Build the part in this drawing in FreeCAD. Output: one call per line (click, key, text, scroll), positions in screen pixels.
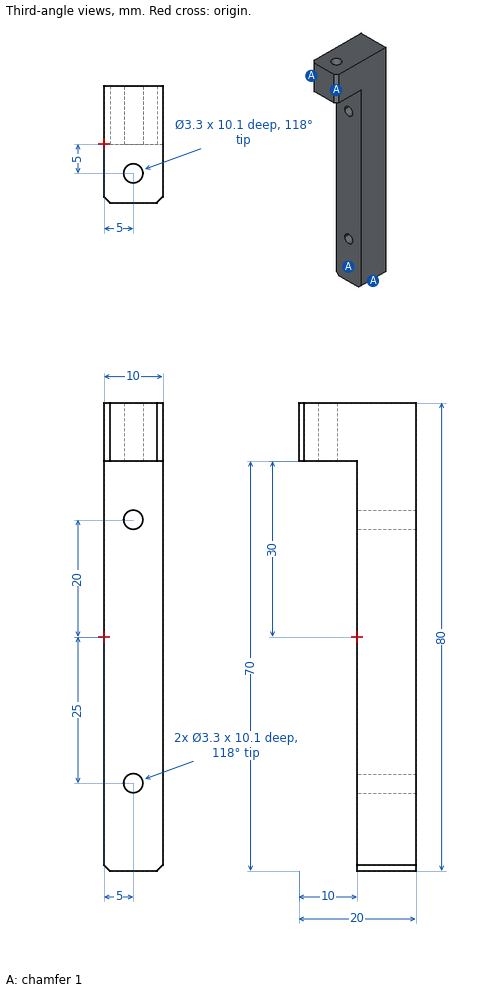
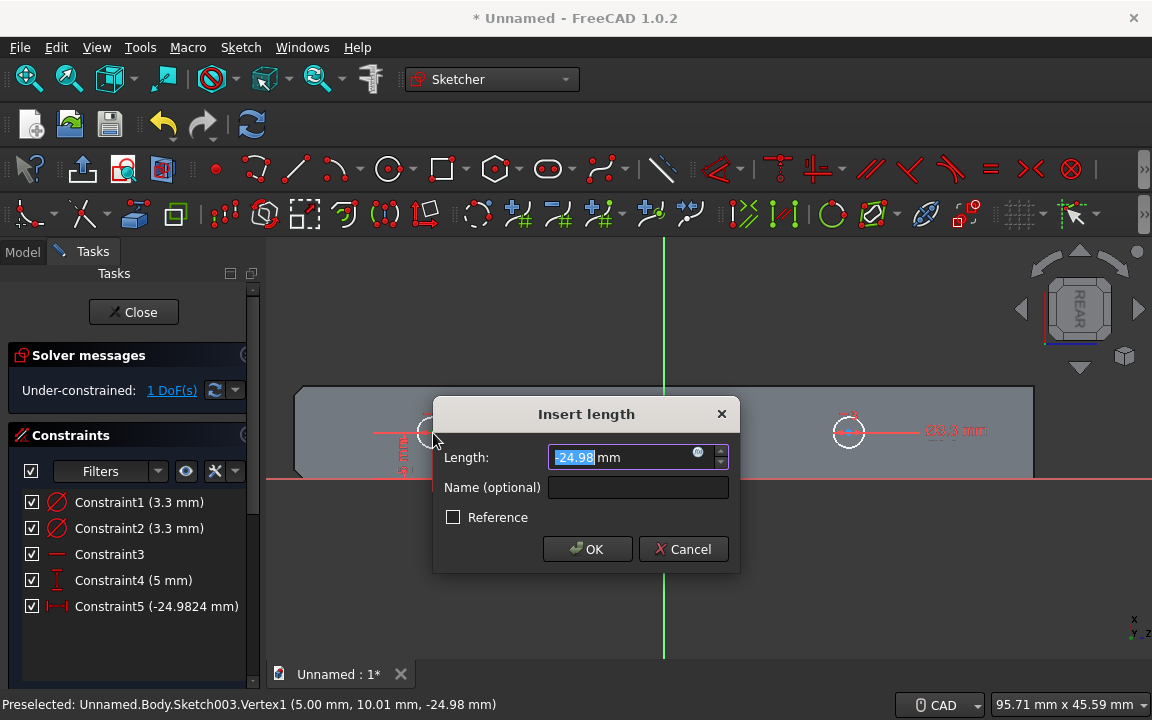
text(-25)
key(Return)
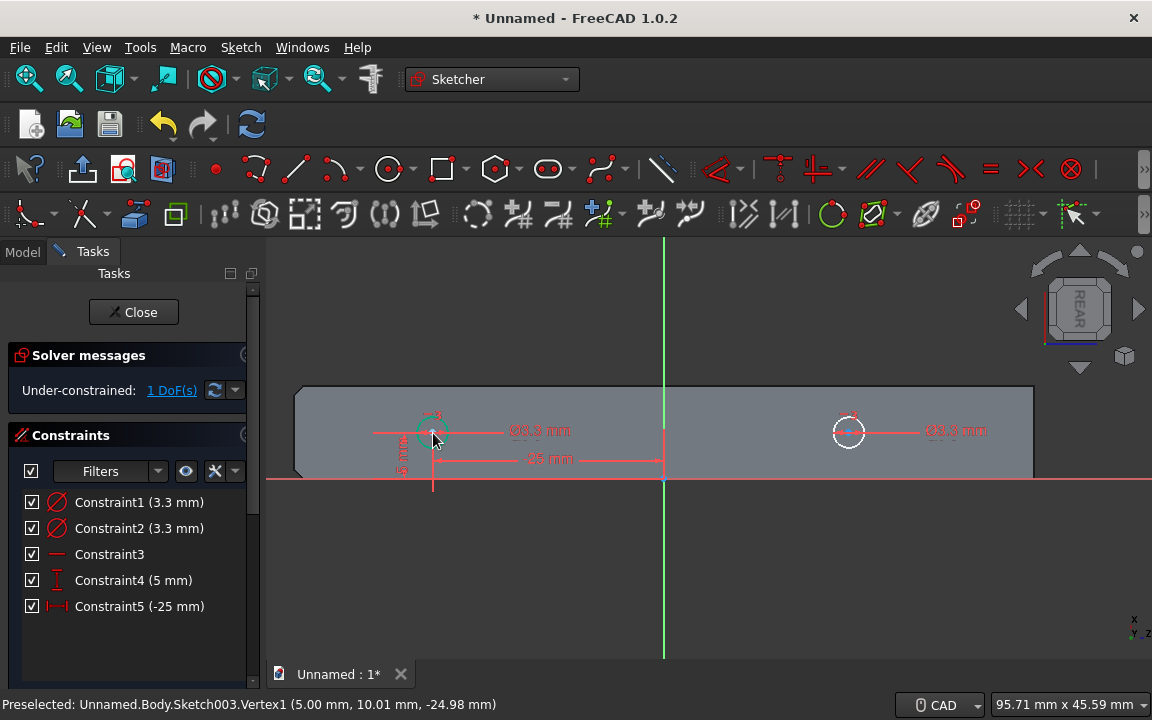
click(849, 433)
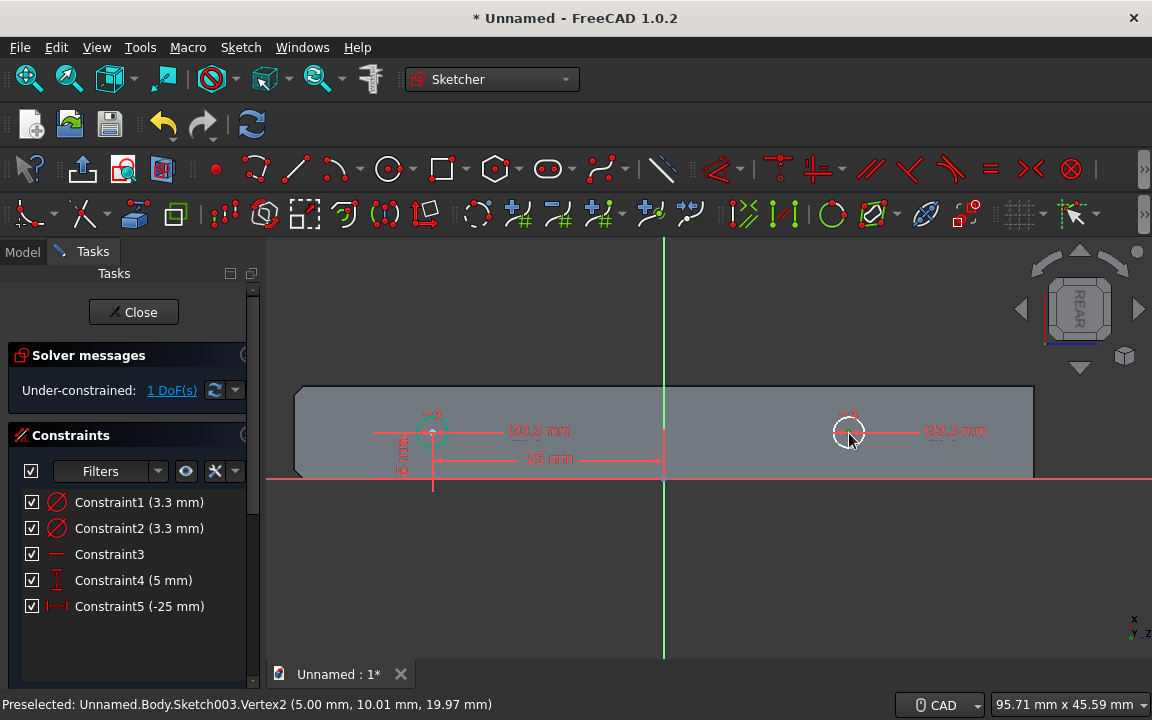
key(l)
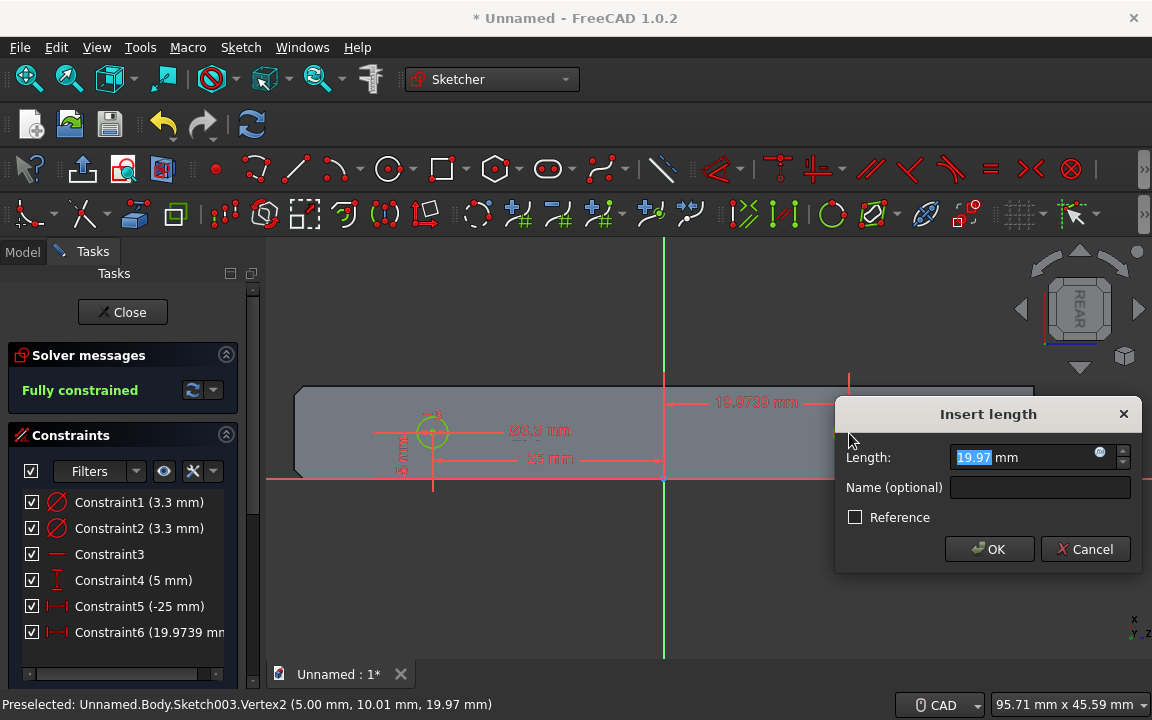
text(20)
key(Return)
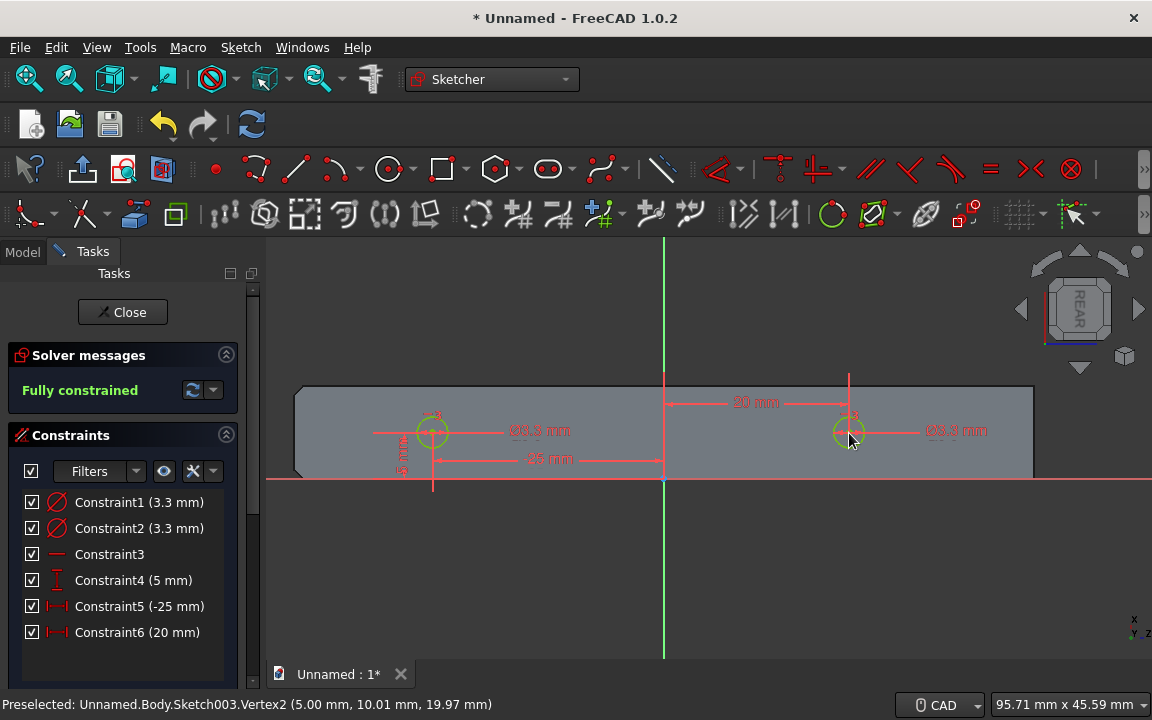
click(123, 312)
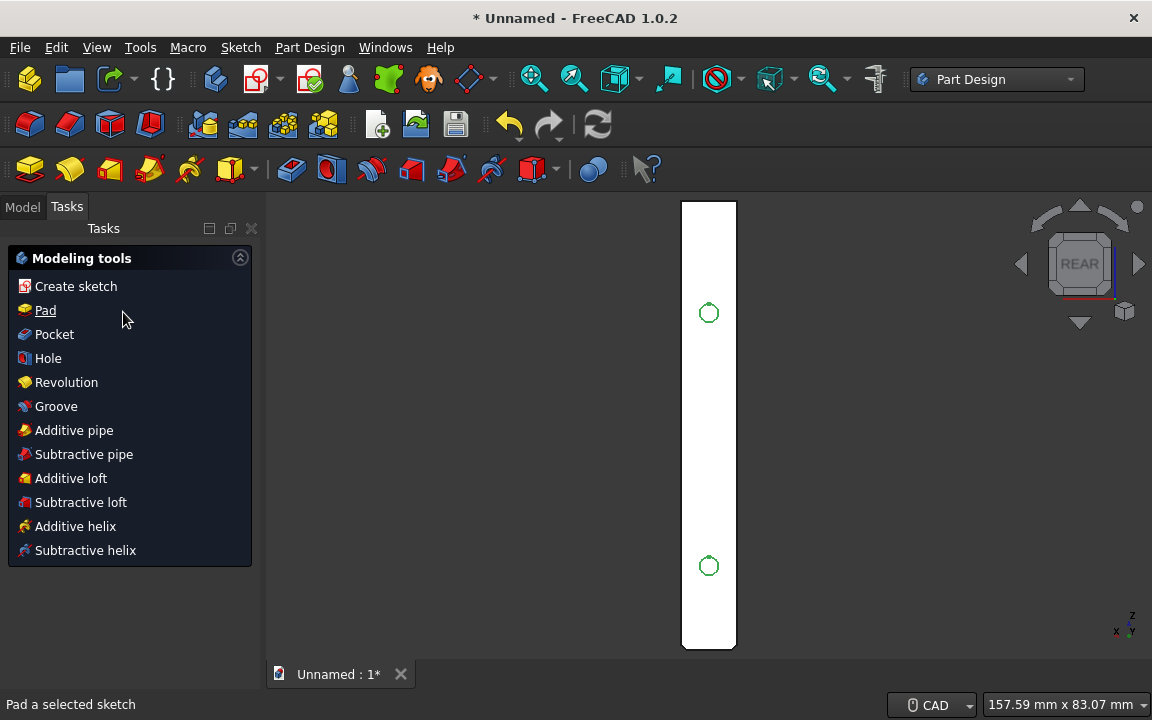
click(332, 170)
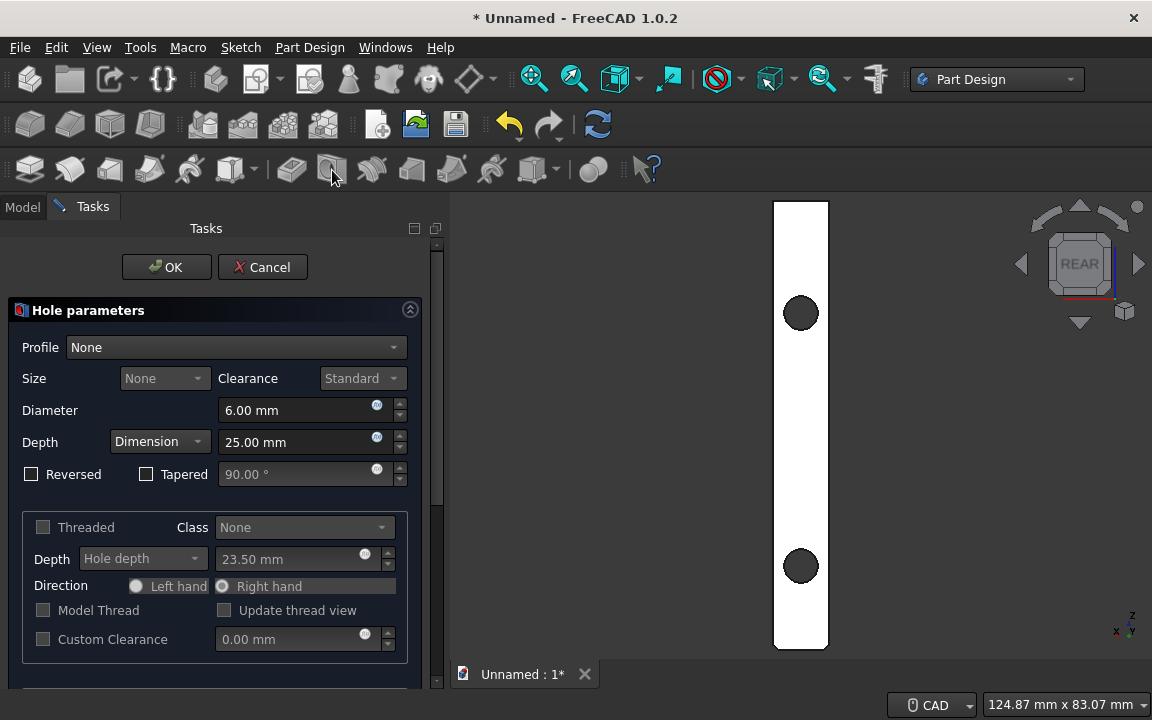
triple_click(305, 410)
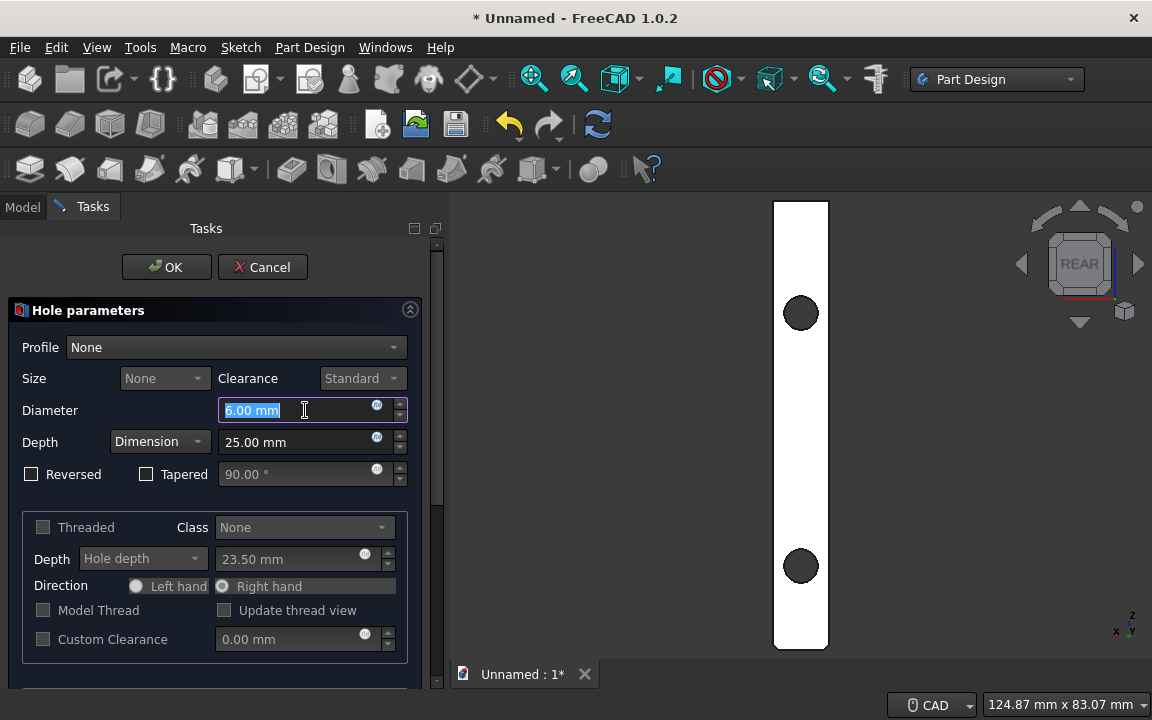
text(3.3)
key(Tab)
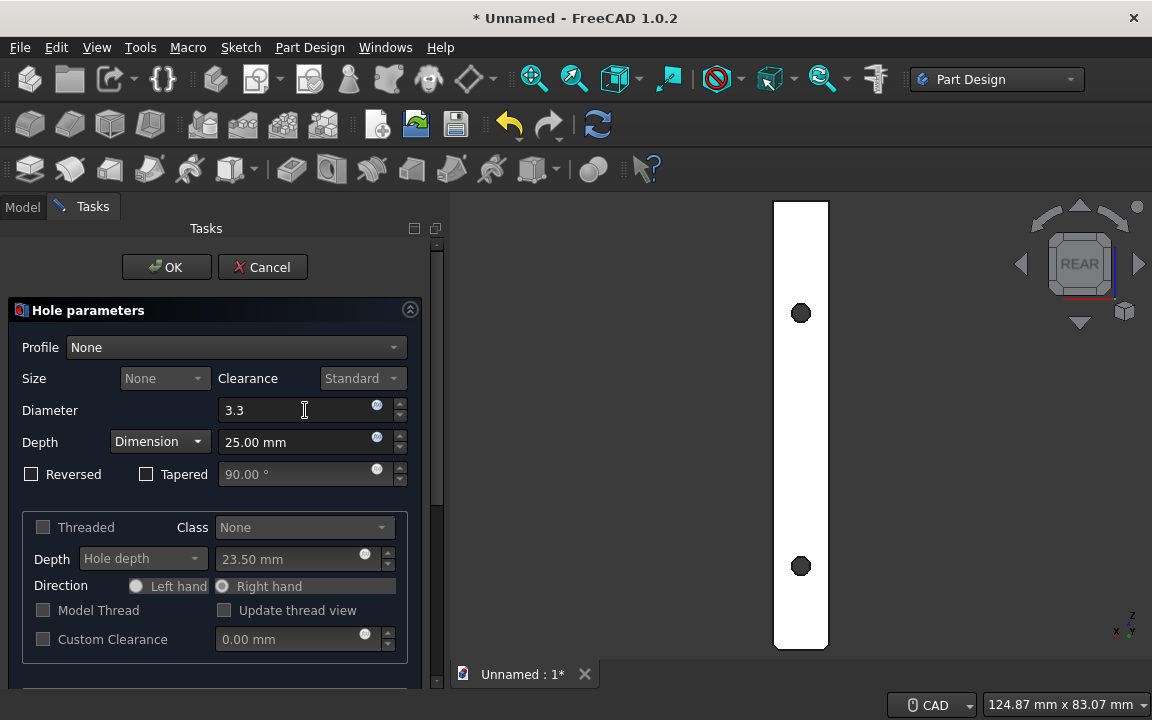
triple_click(305, 442)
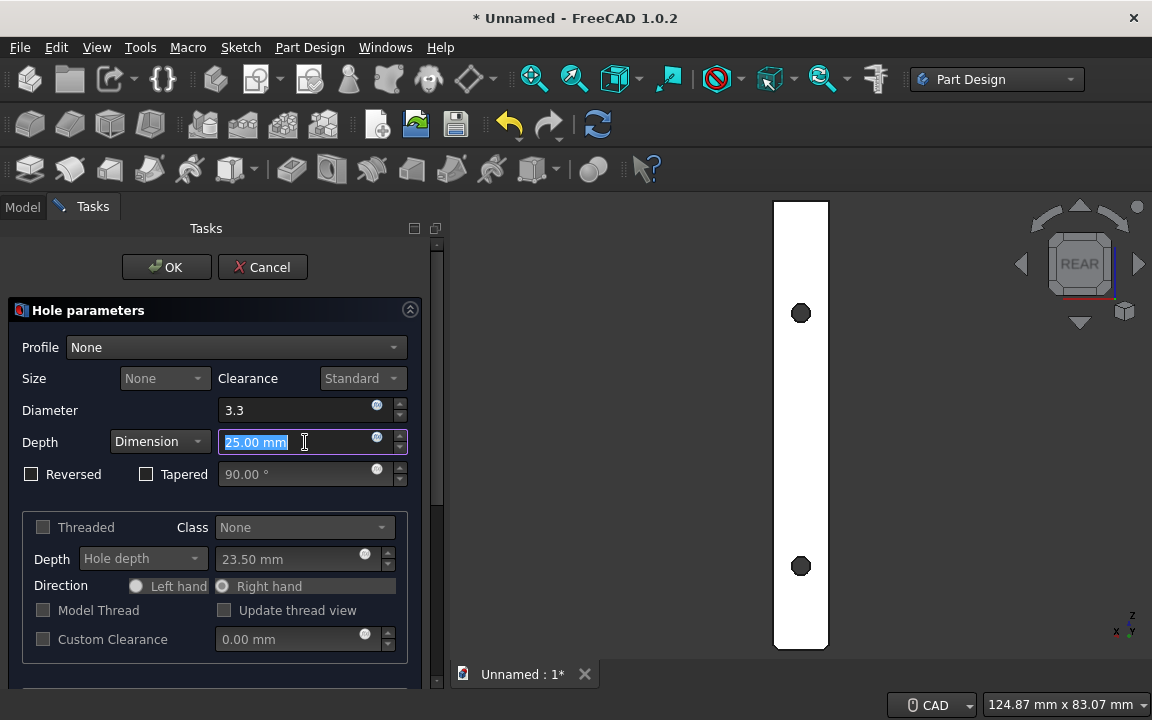
text(10.1)
key(Tab)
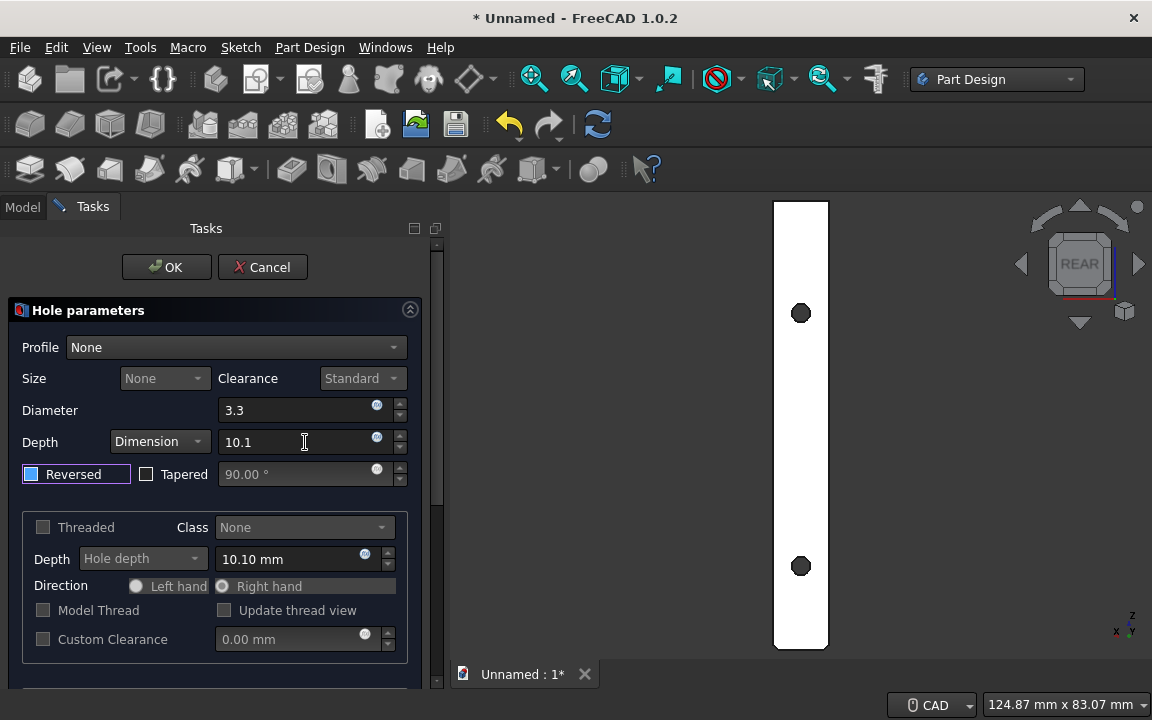
click(167, 267)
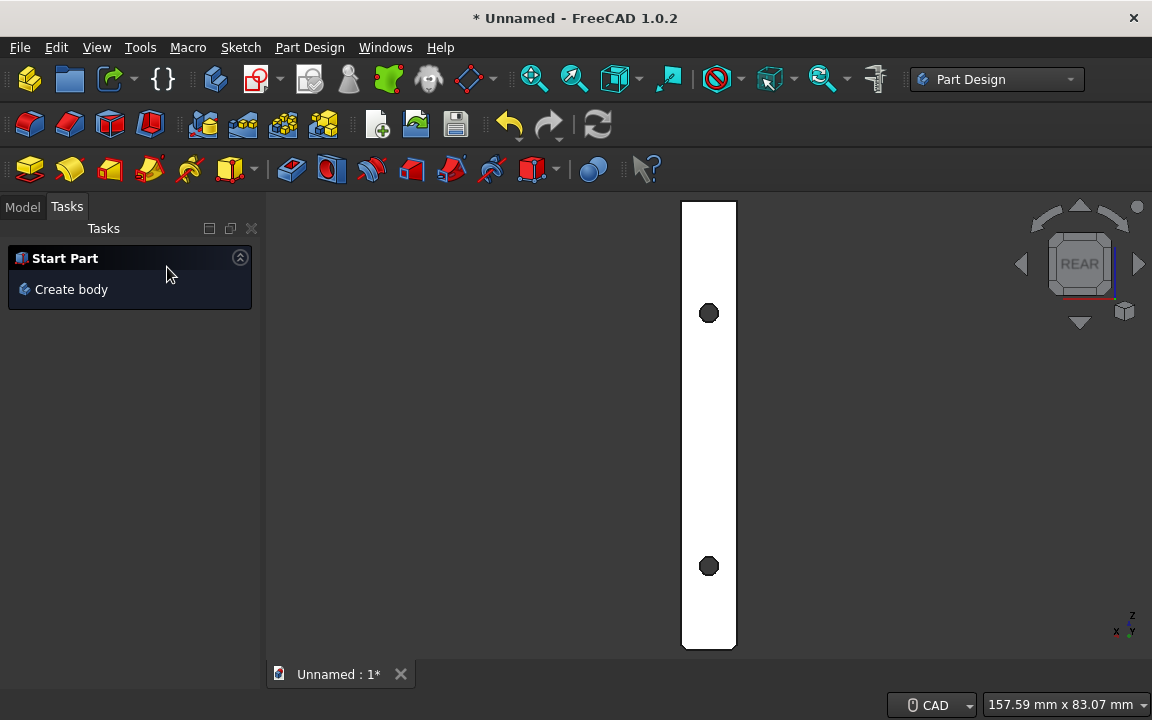
key(0)